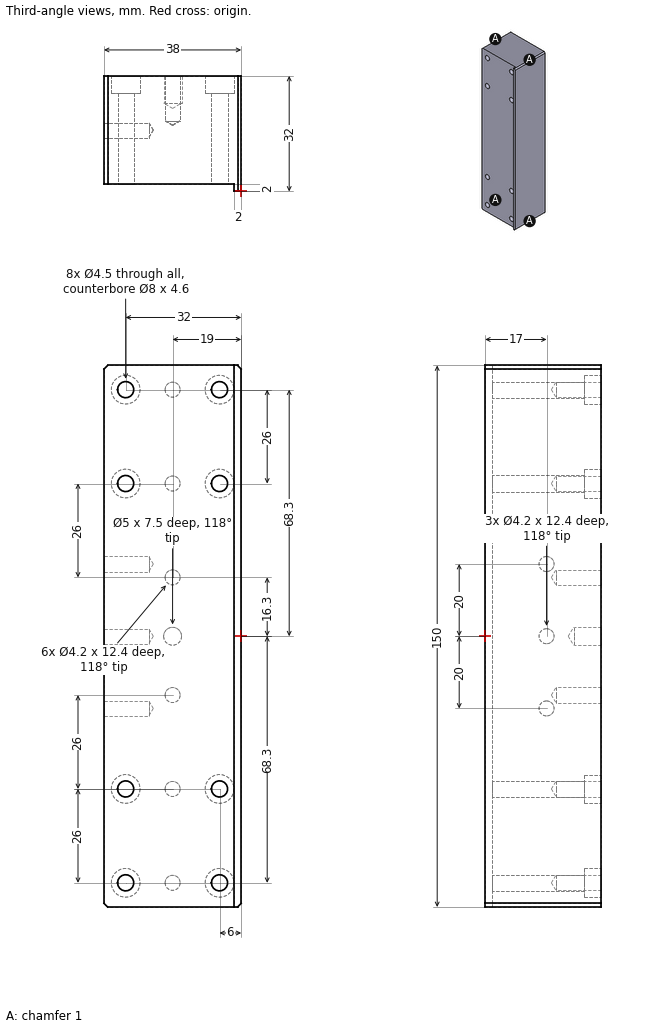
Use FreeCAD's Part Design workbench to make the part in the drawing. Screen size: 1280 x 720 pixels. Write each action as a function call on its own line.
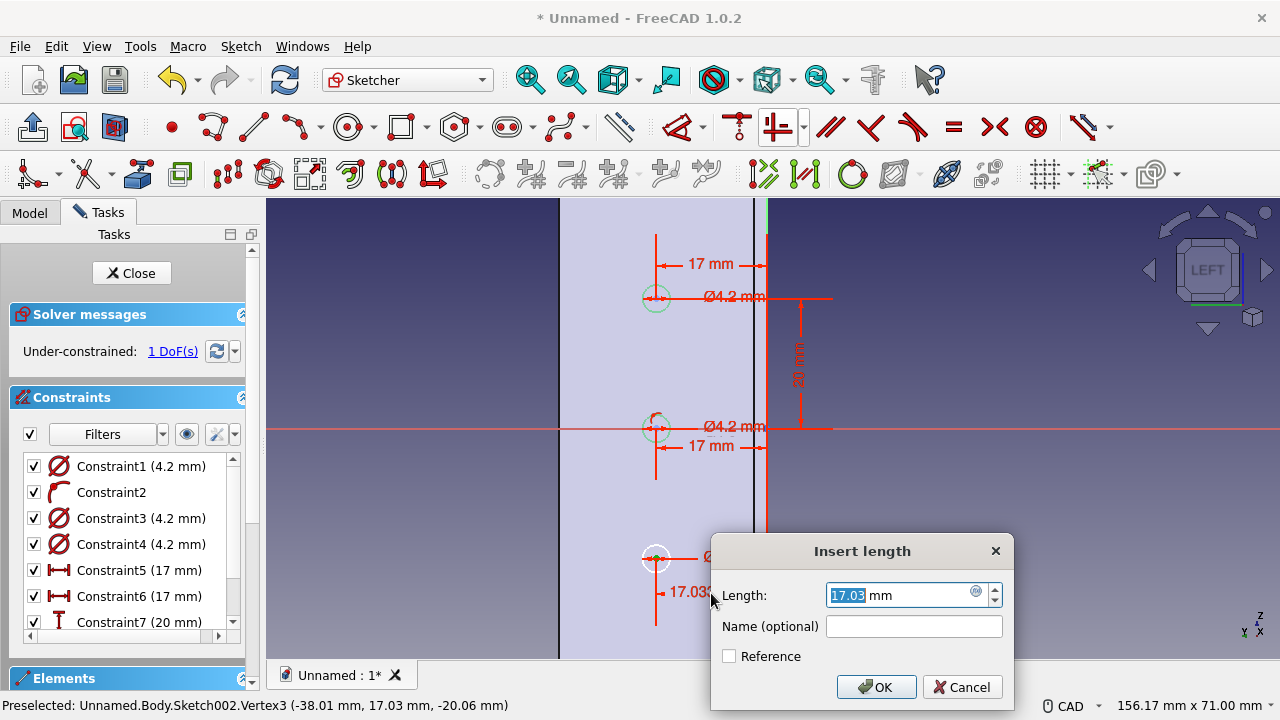
text(17)
key(Return)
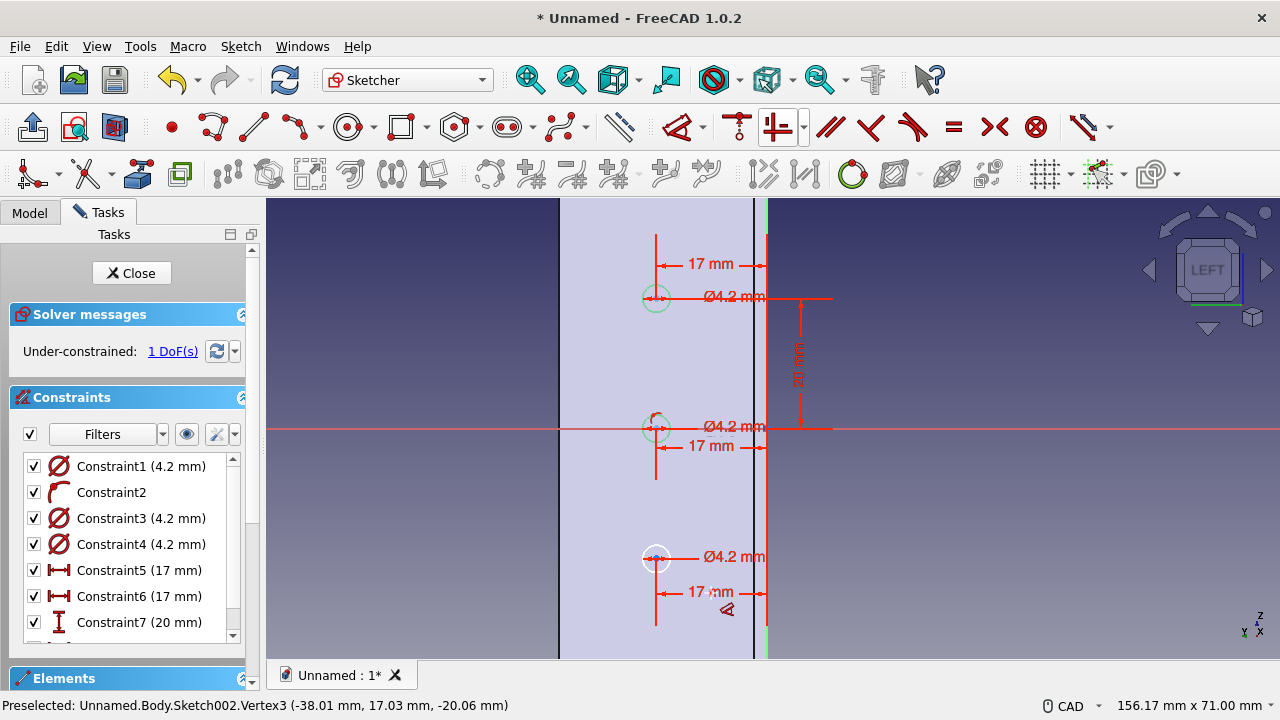
click(656, 559)
click(801, 494)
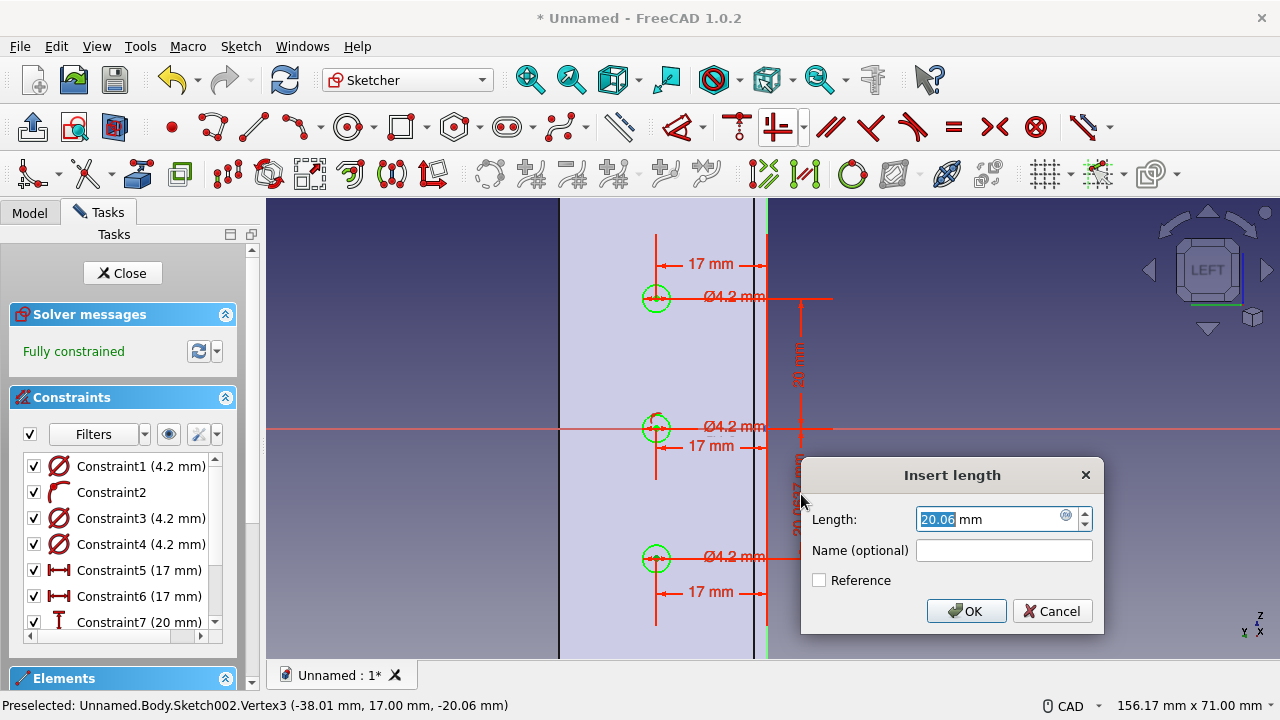
text(20)
key(Return)
key(Escape)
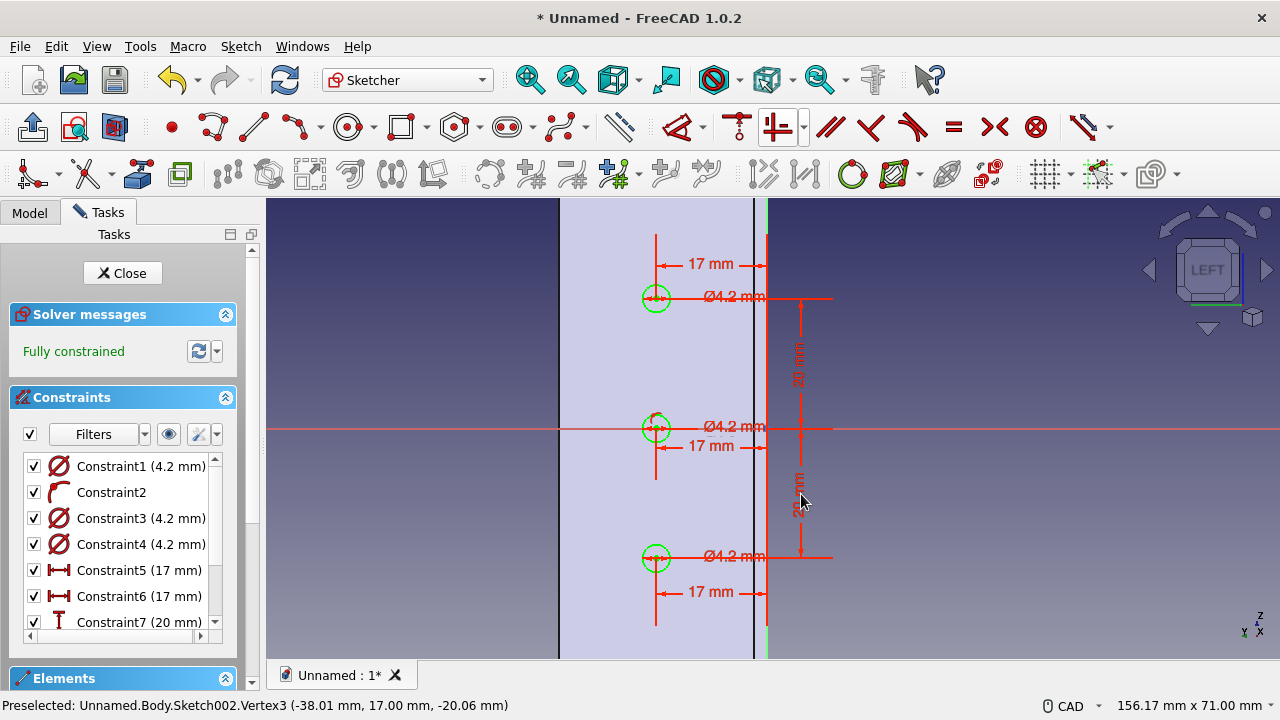
click(123, 273)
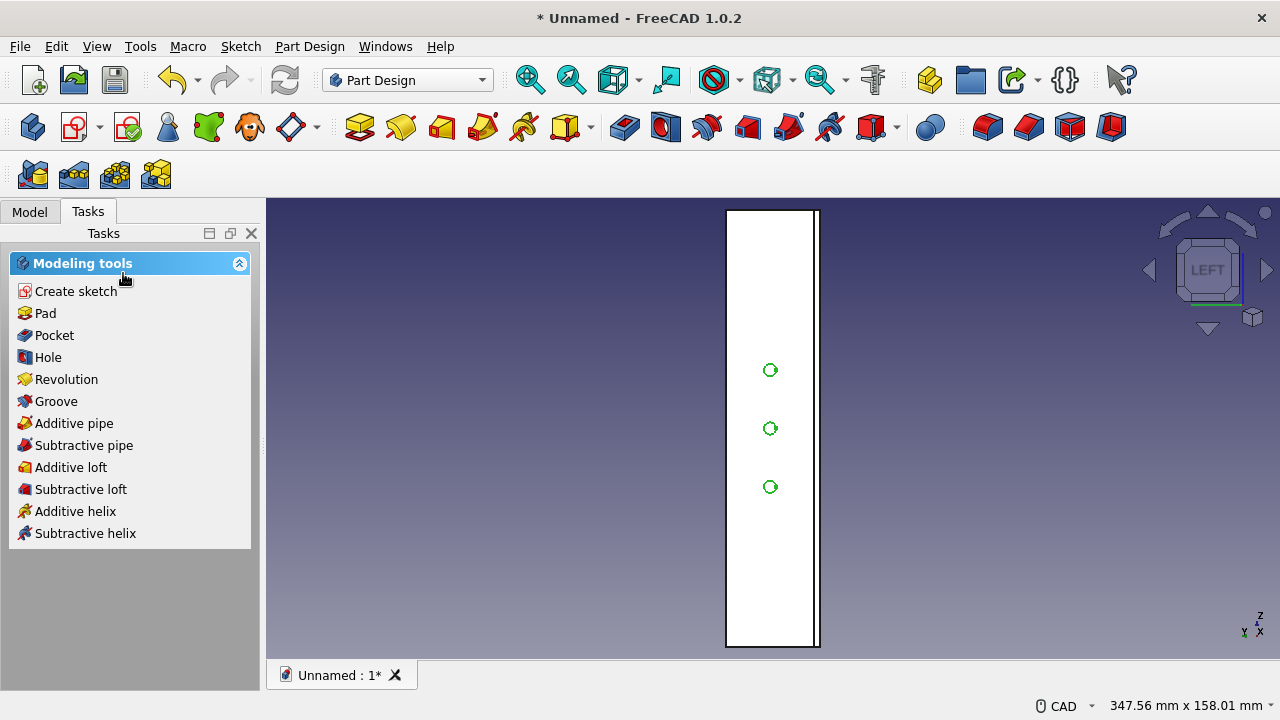
click(666, 128)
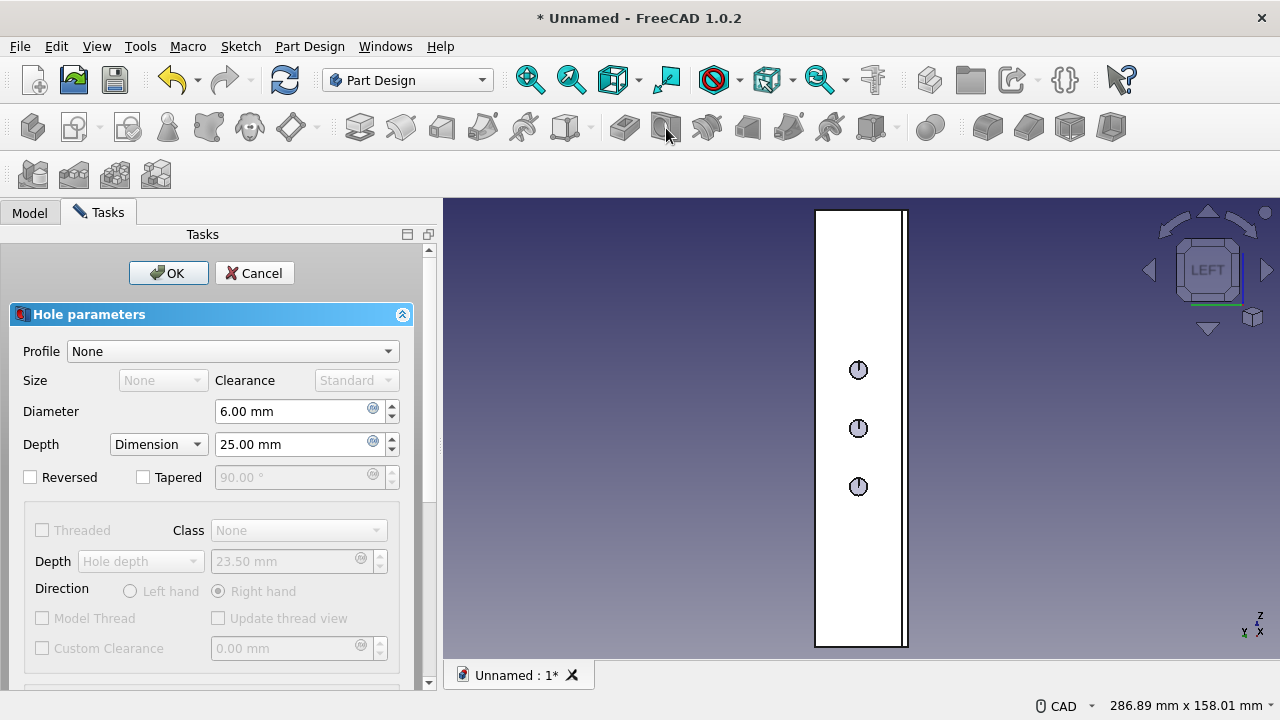
triple_click(300, 412)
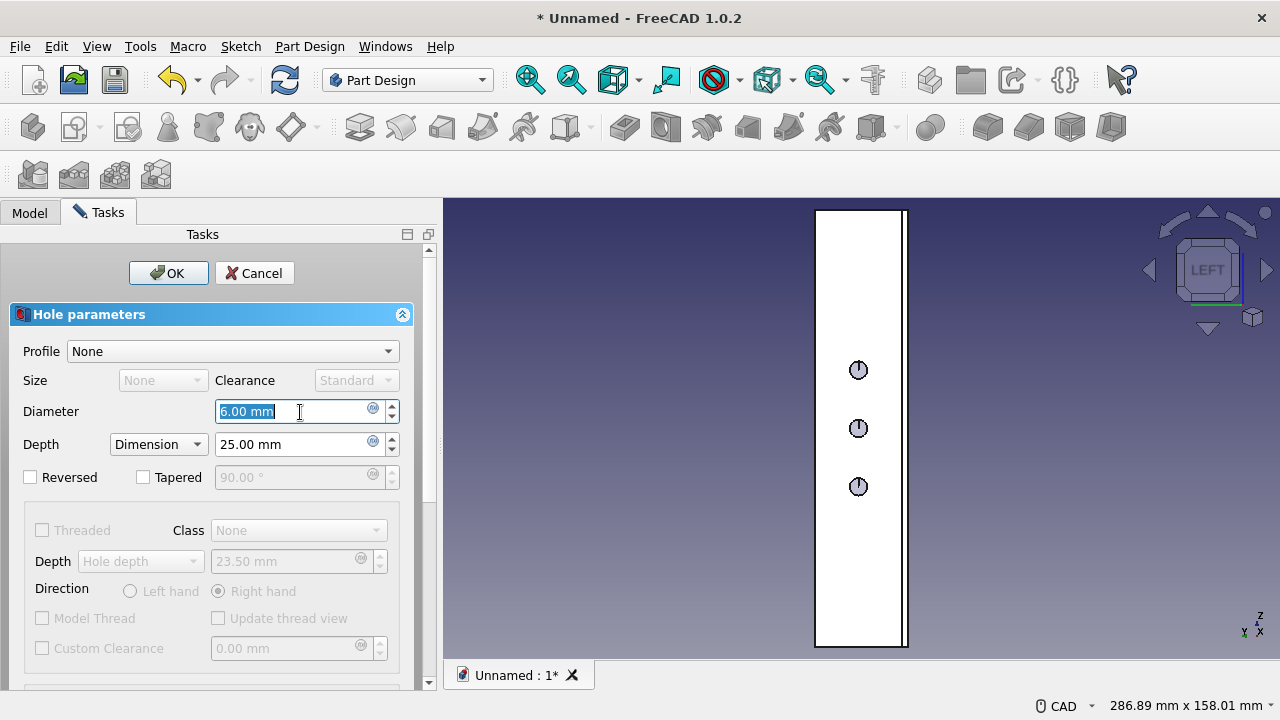
text(4.2)
key(Tab)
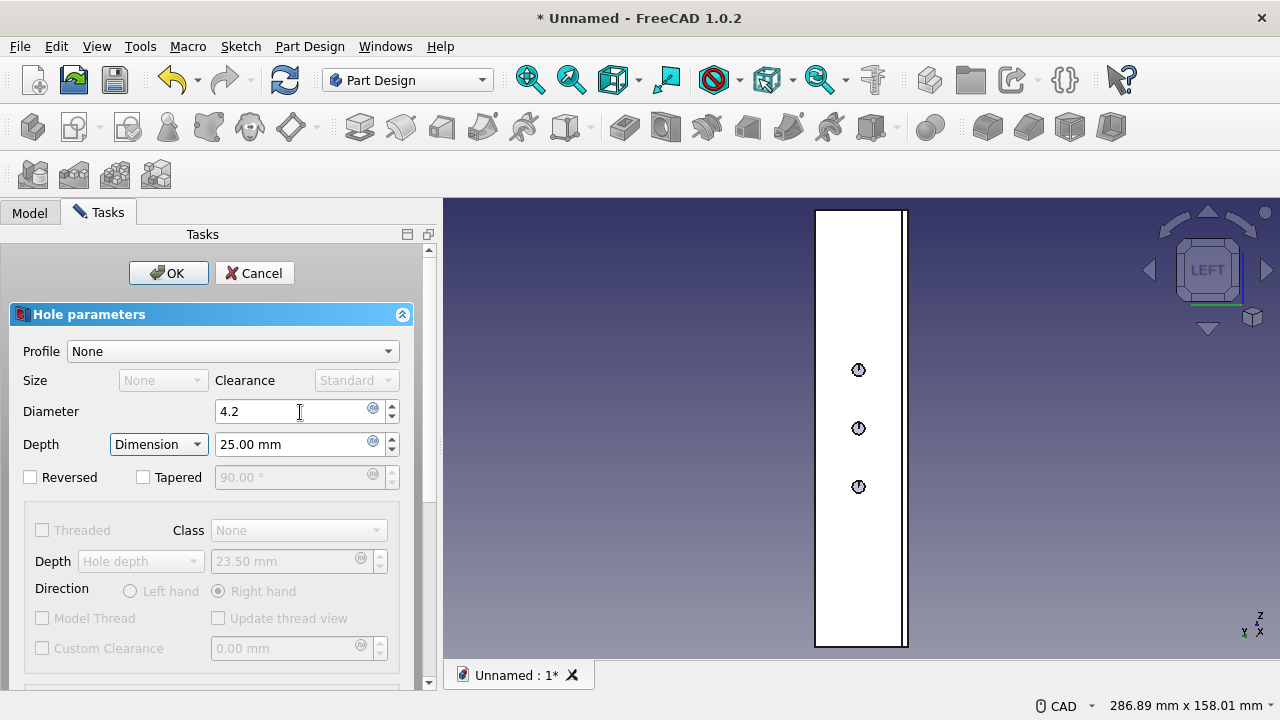
triple_click(300, 444)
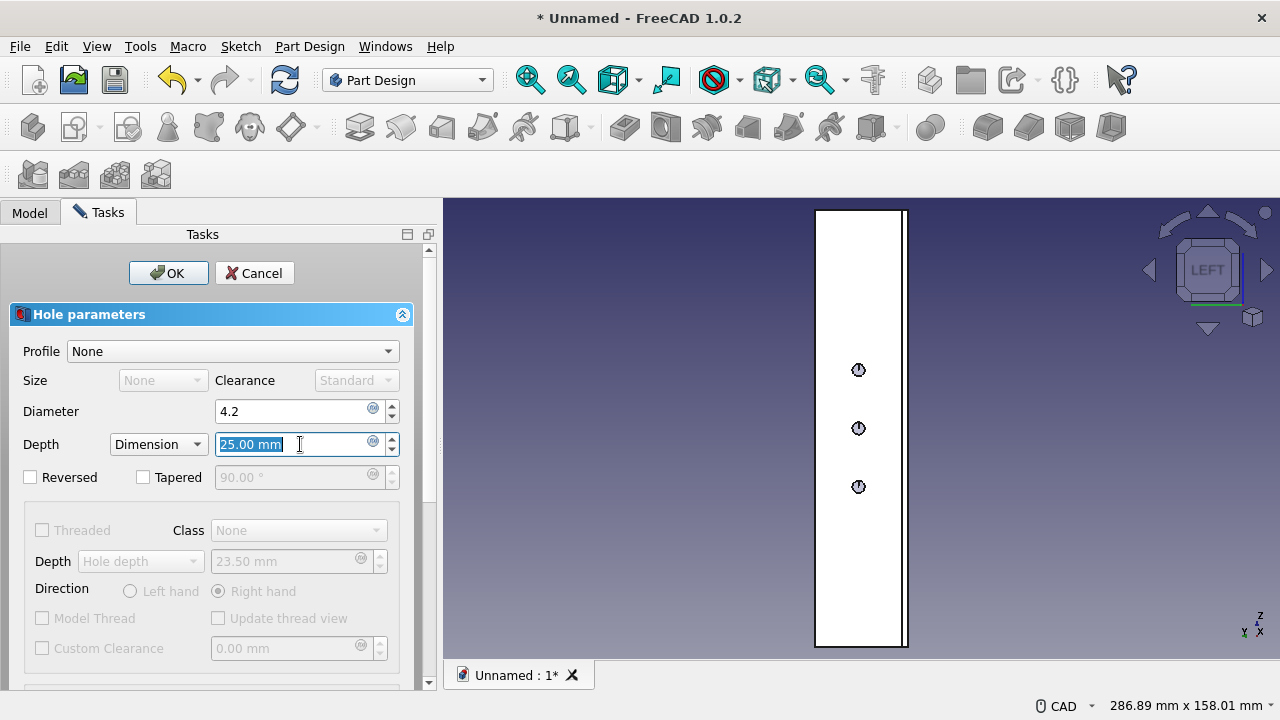
text(12.4)
key(Tab)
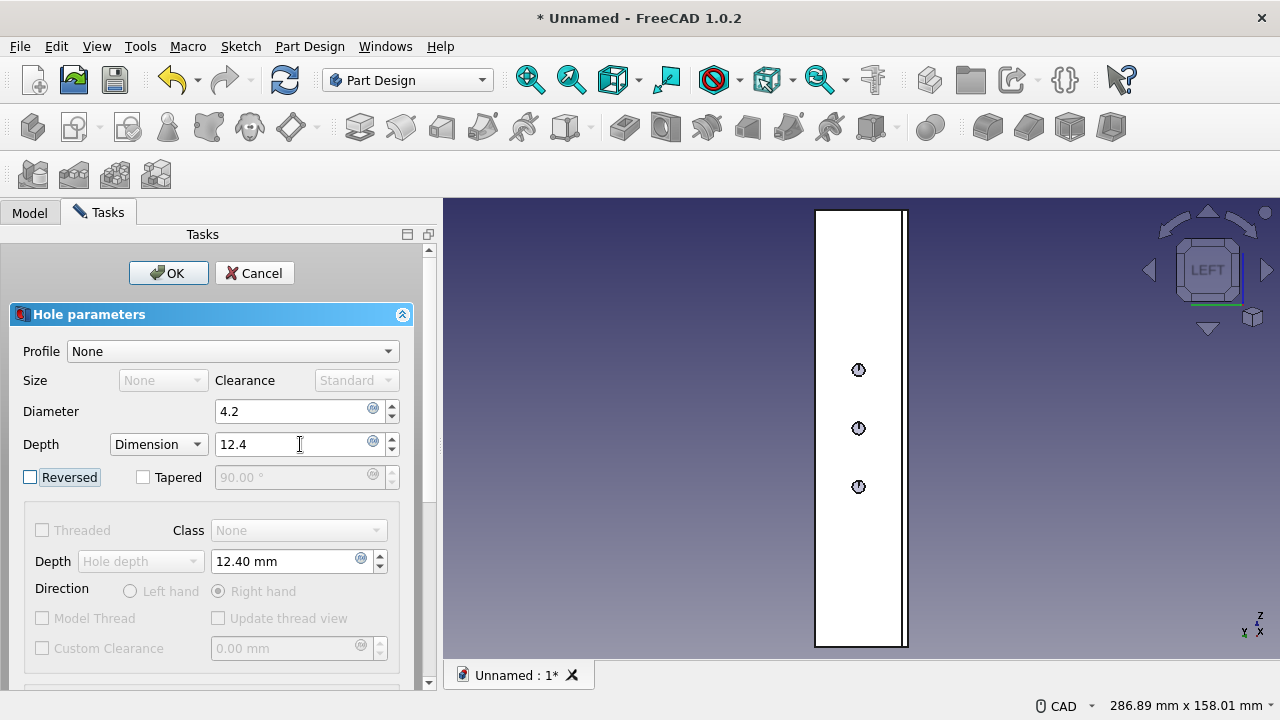
click(169, 273)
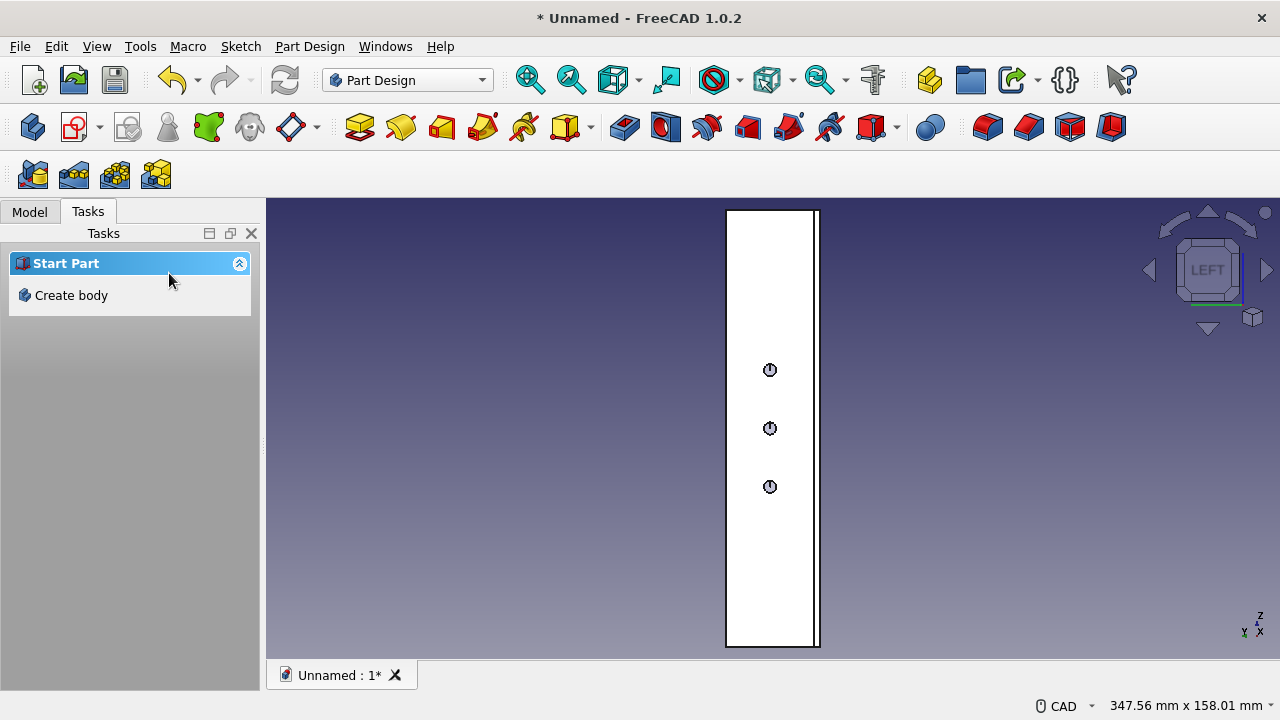
key(4)